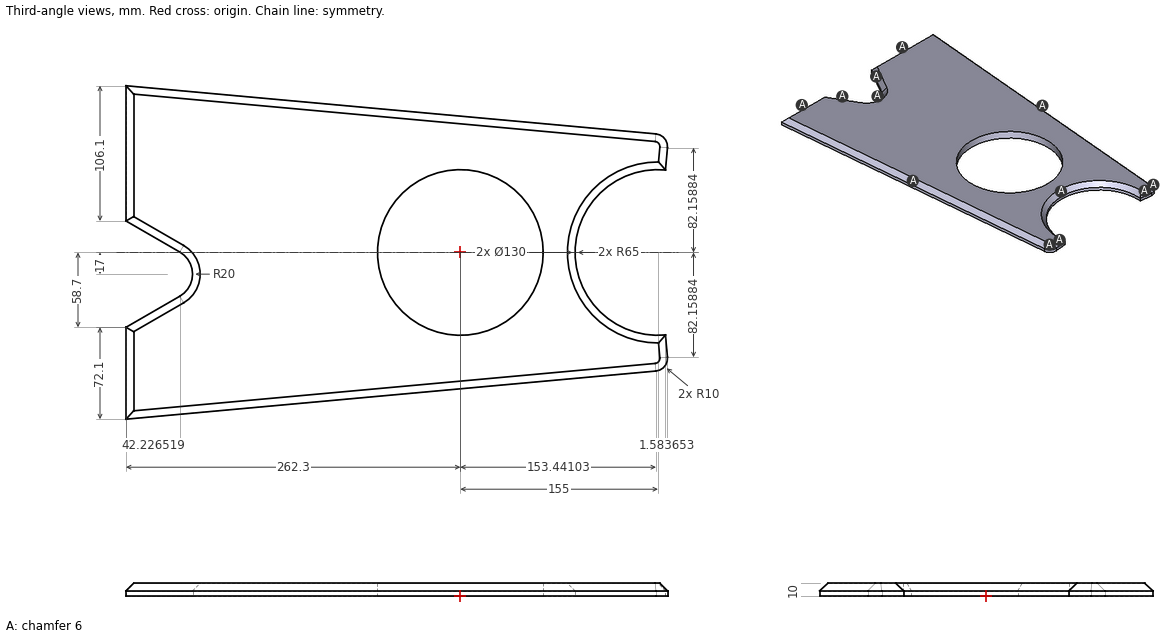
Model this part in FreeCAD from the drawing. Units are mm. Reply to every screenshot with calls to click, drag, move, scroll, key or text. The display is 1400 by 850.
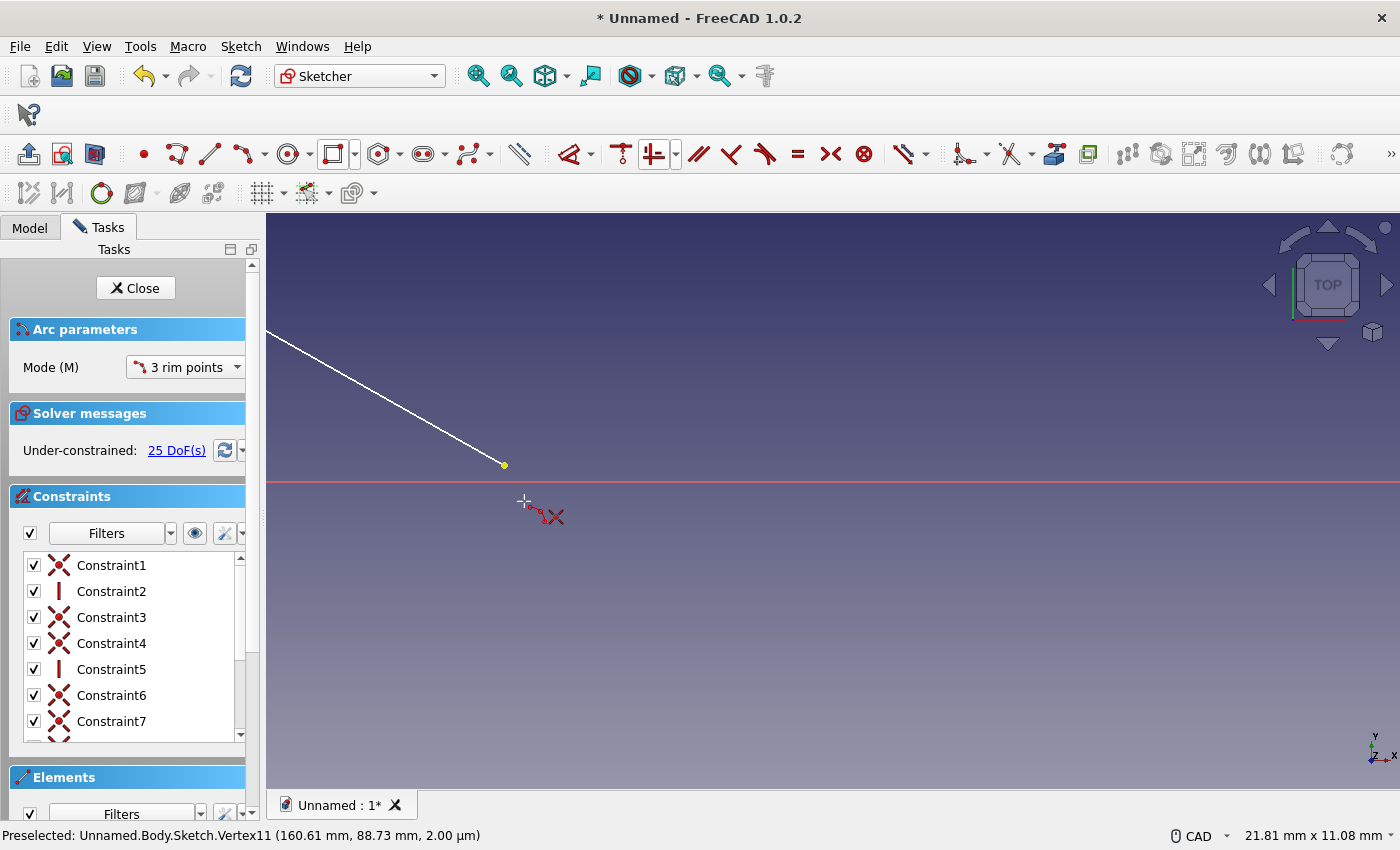
click(504, 466)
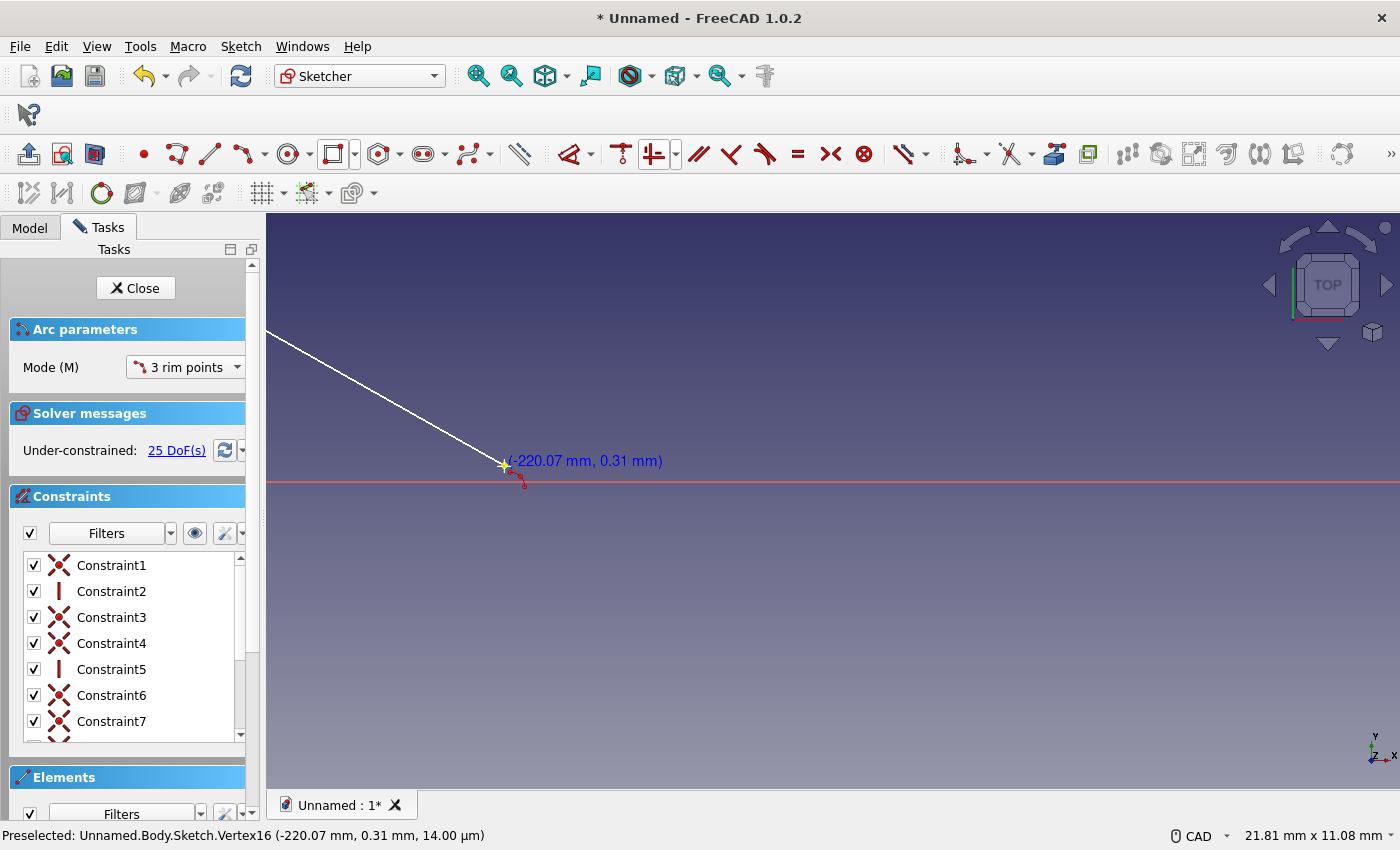
scroll(468, 502, down, 17)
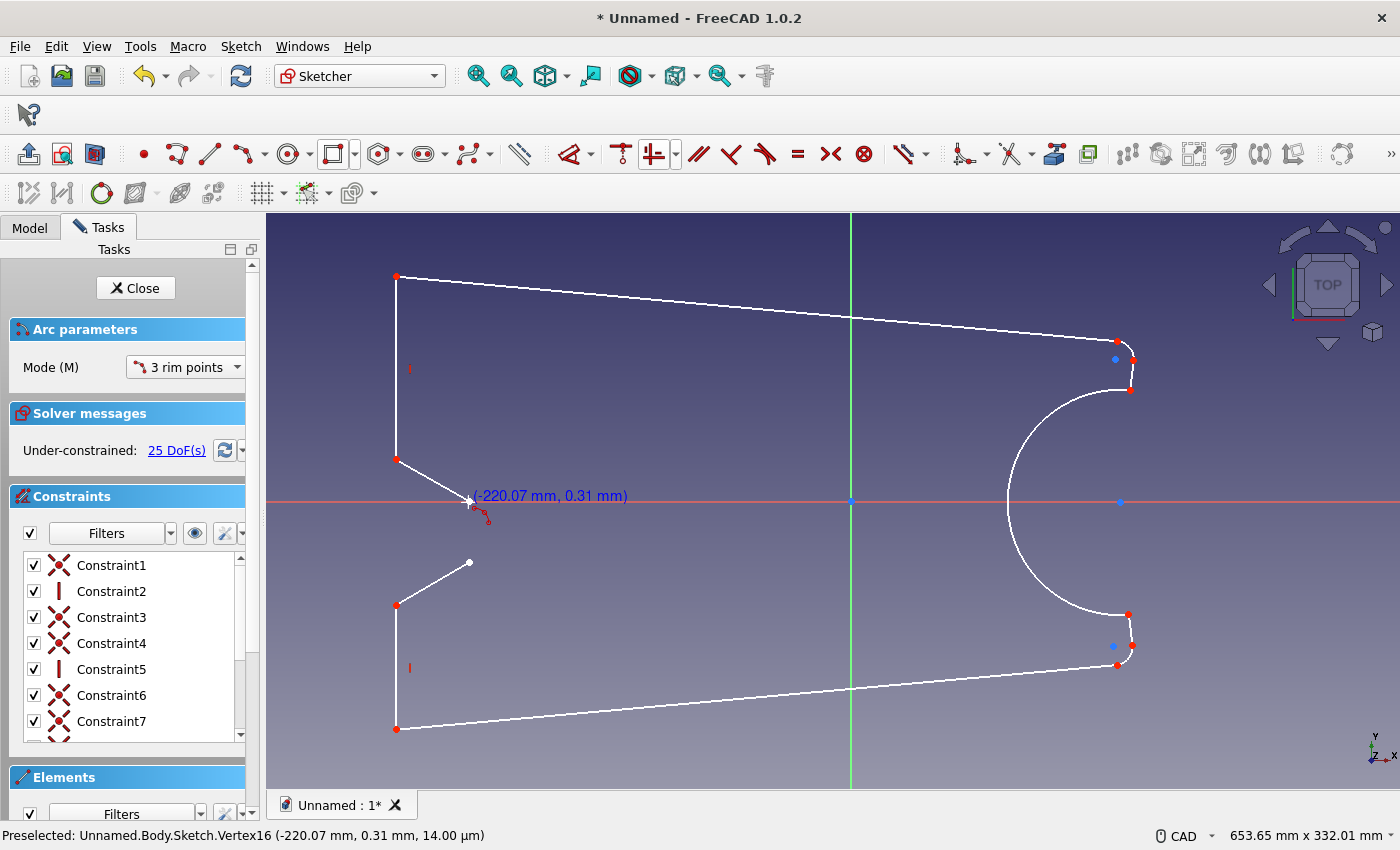
click(469, 562)
click(487, 531)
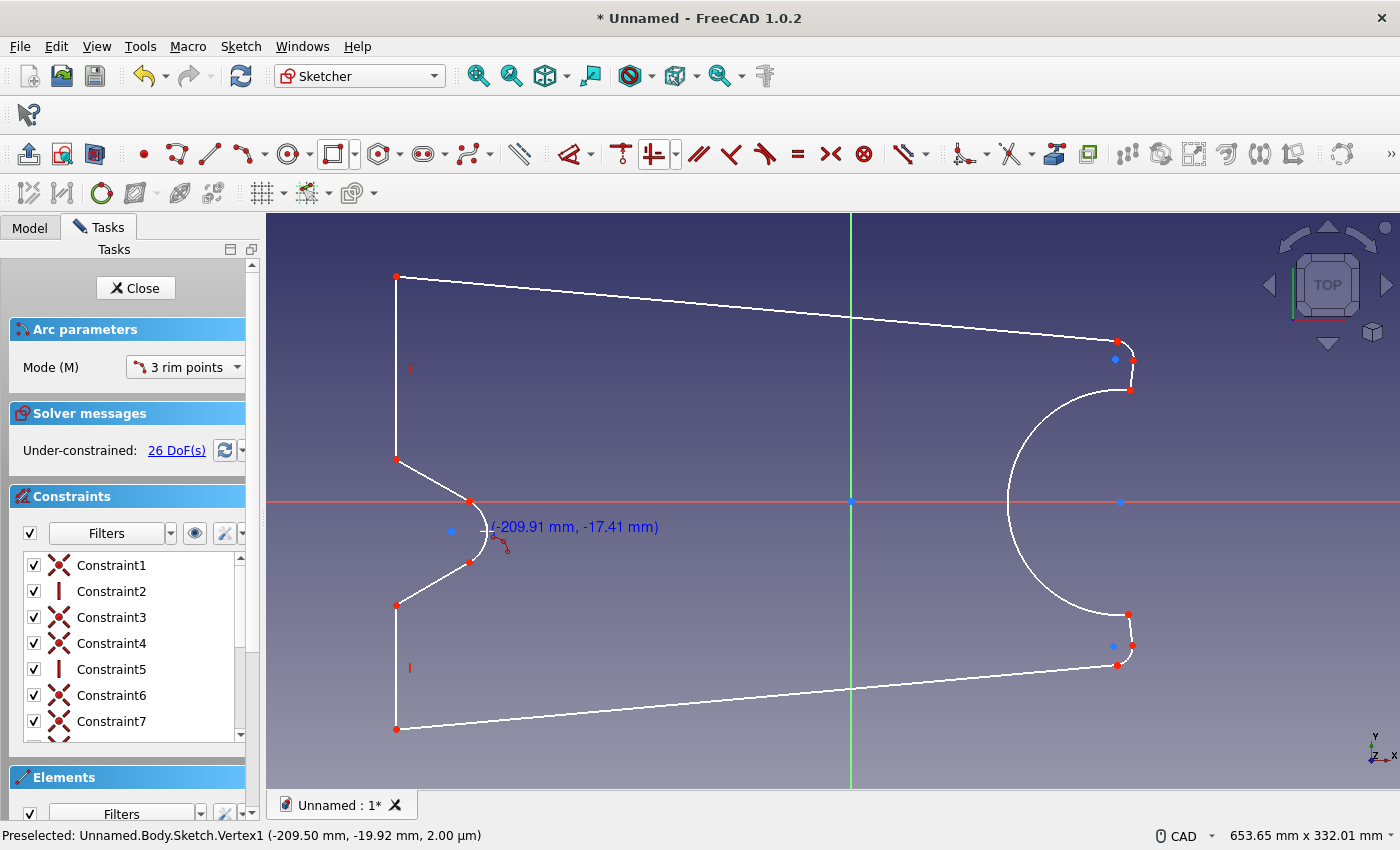
click(288, 154)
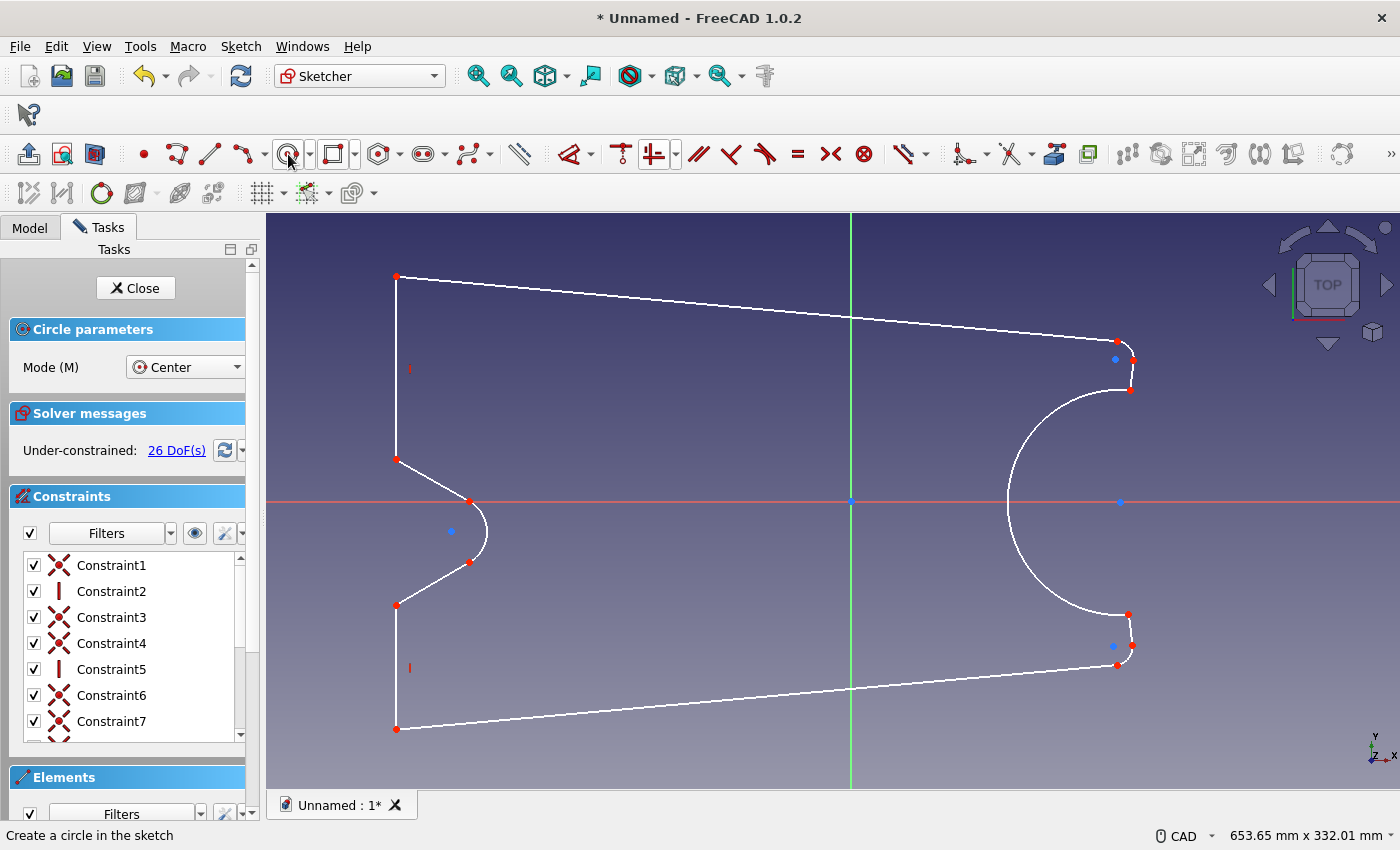
click(851, 502)
click(931, 422)
key(Escape)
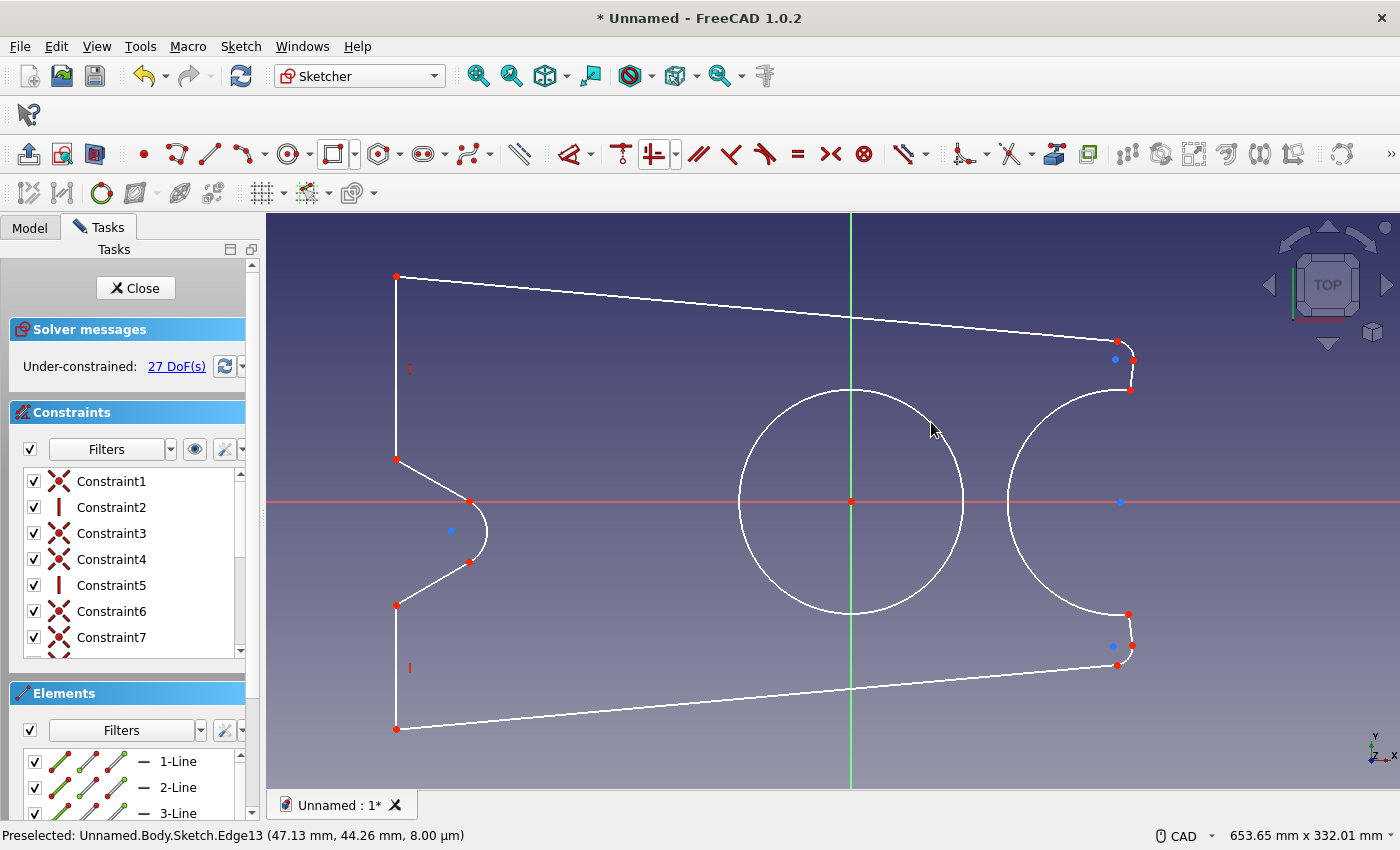
click(447, 575)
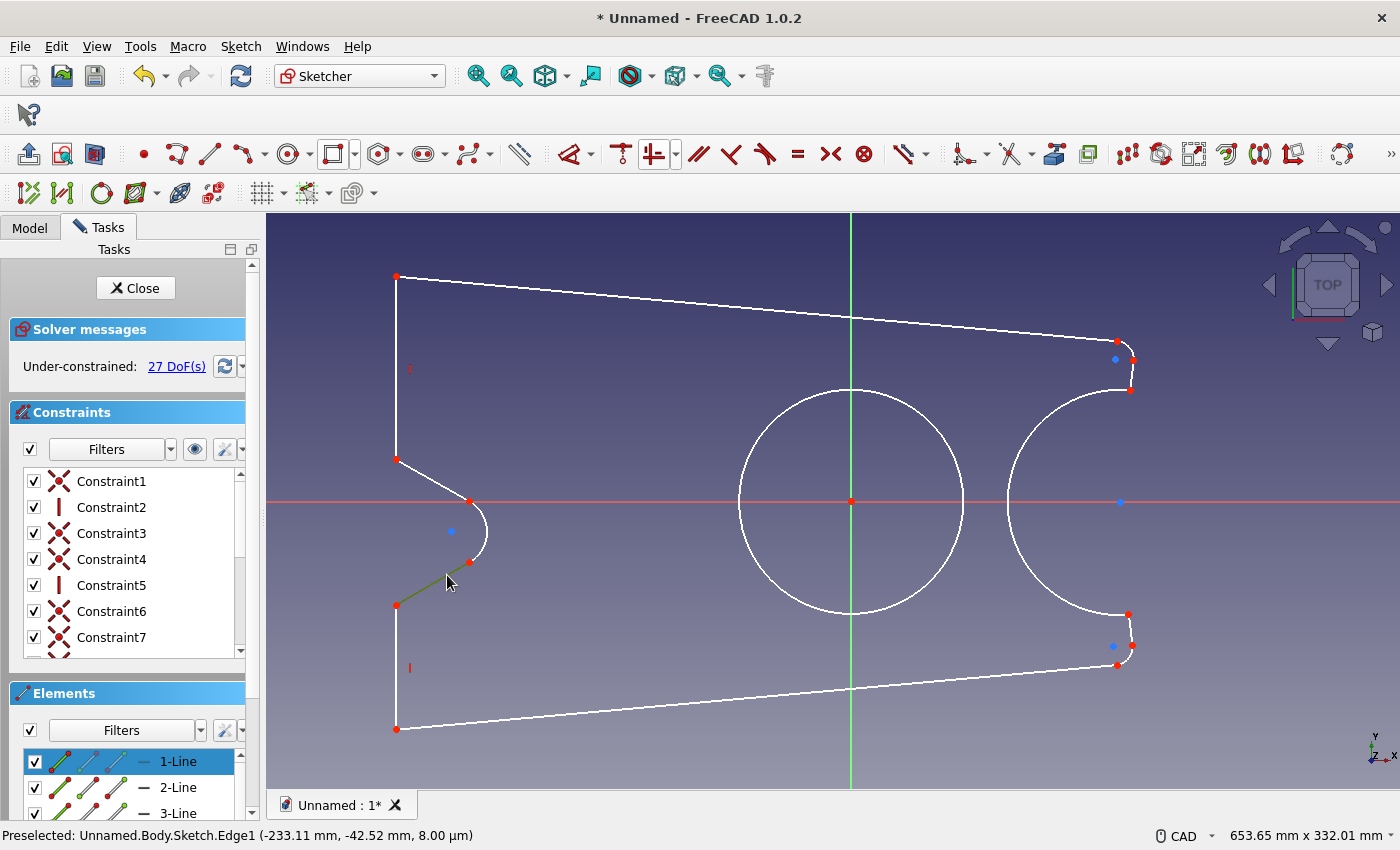
click(484, 546)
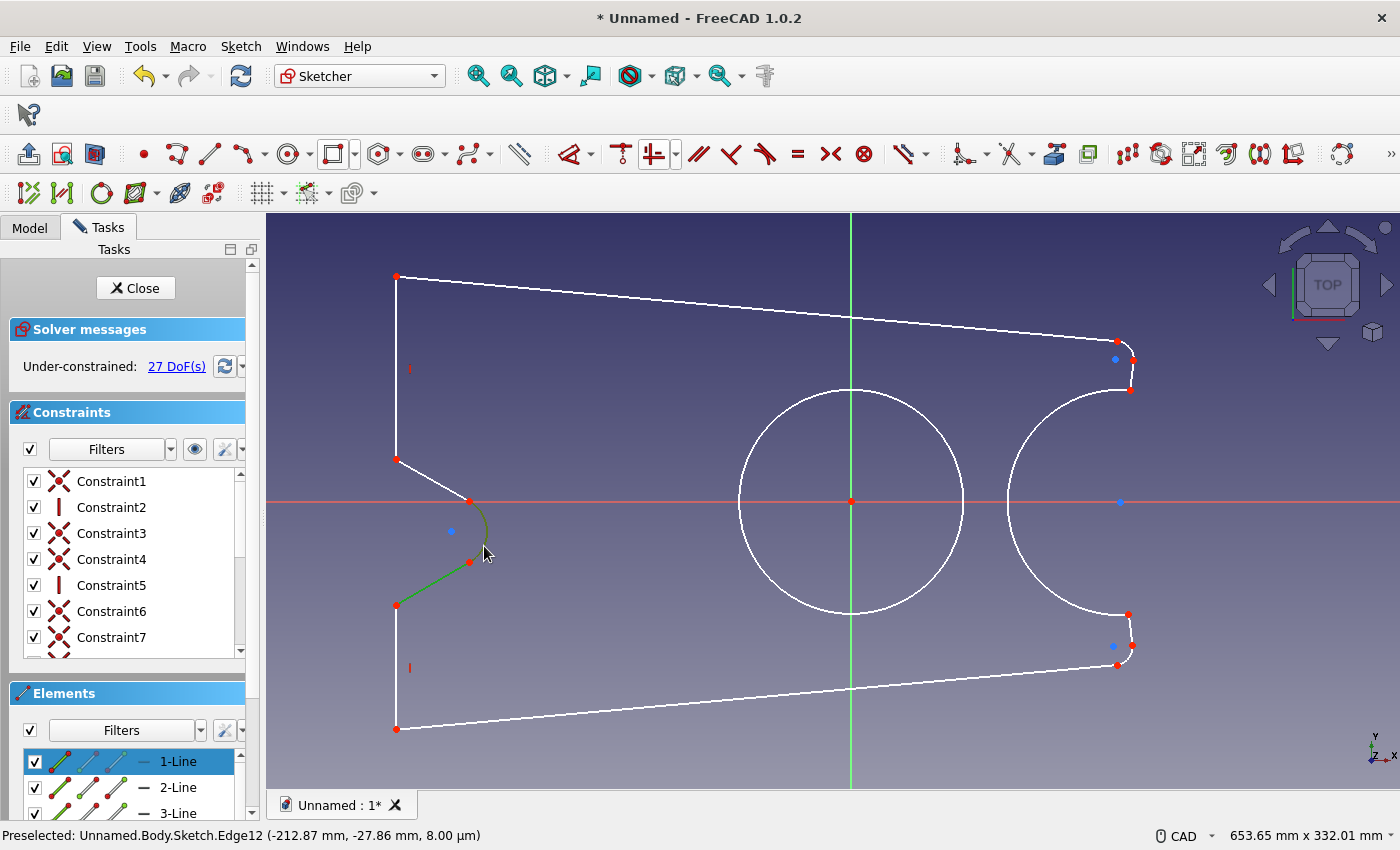
click(765, 154)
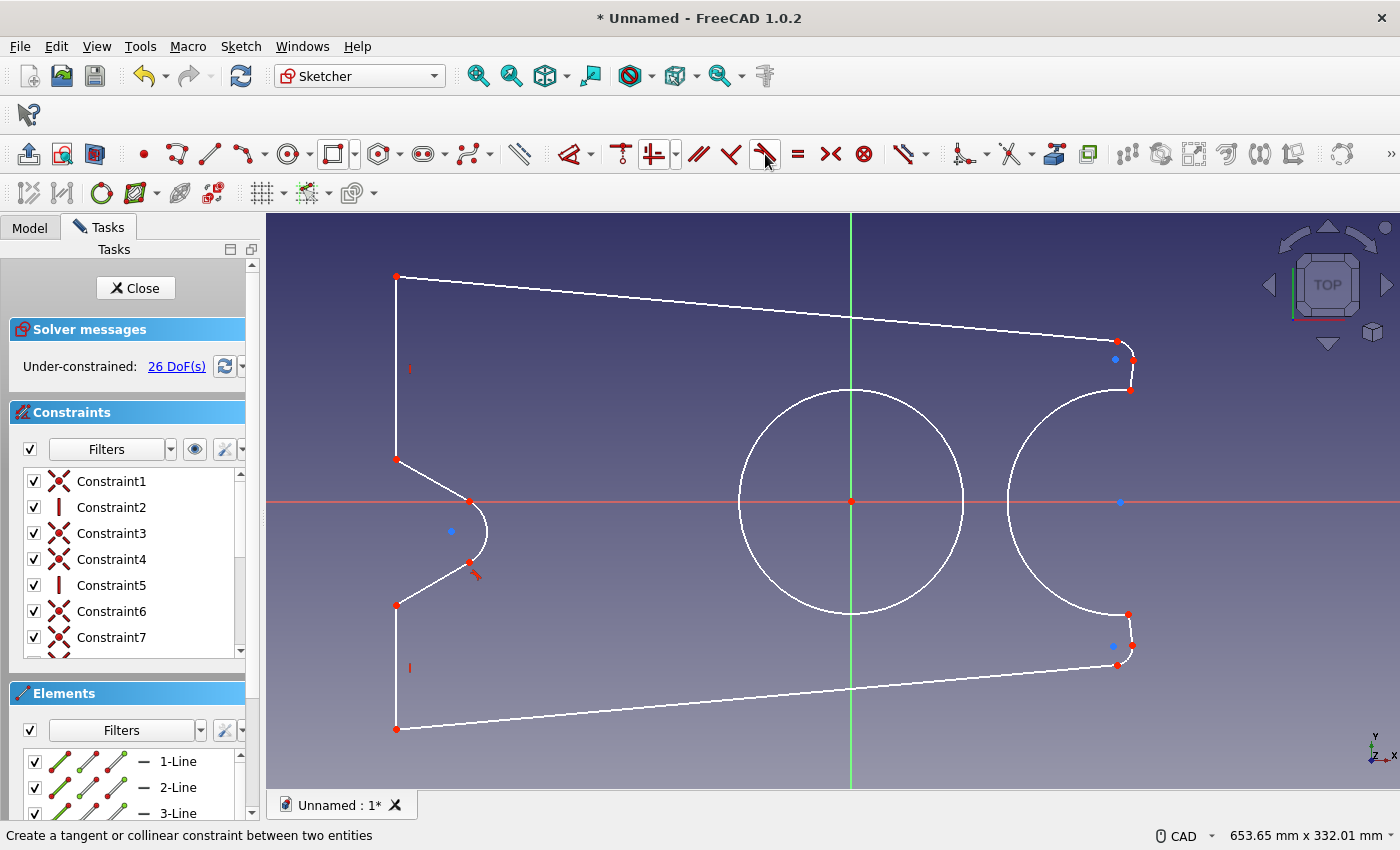
click(613, 710)